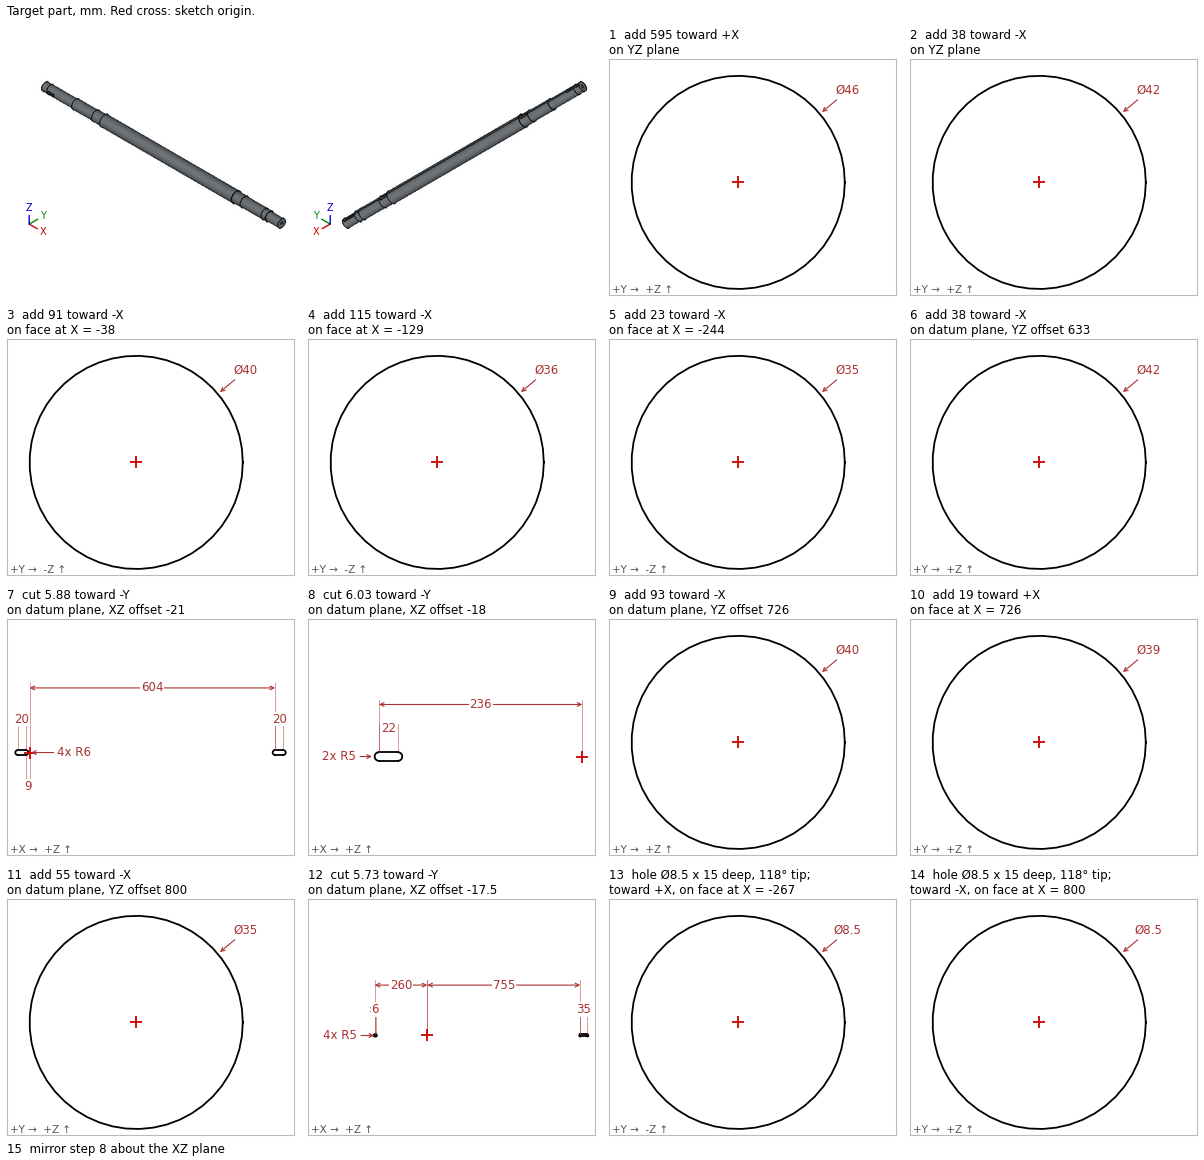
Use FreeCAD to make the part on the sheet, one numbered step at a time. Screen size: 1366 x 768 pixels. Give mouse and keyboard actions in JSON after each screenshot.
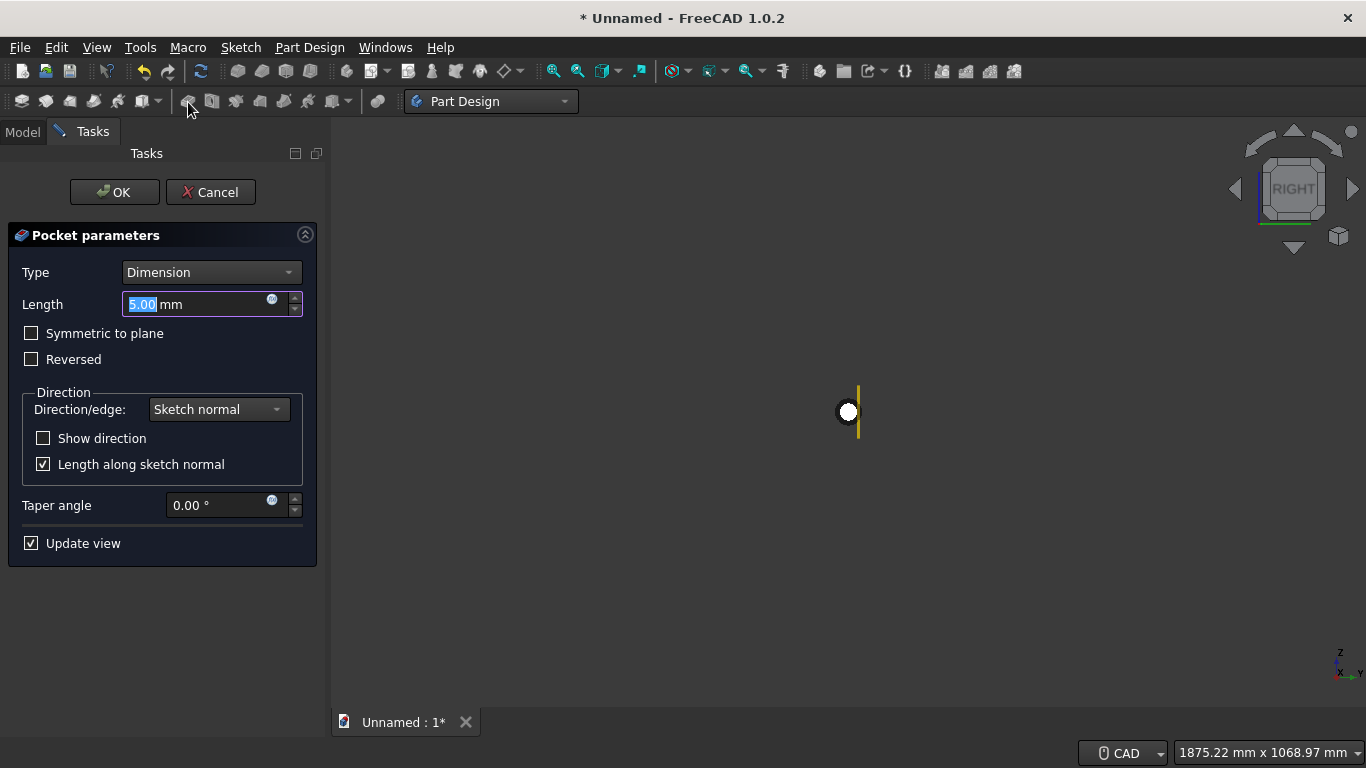
{"action": "type", "text": "5.73"}
{"action": "key", "text": "Tab"}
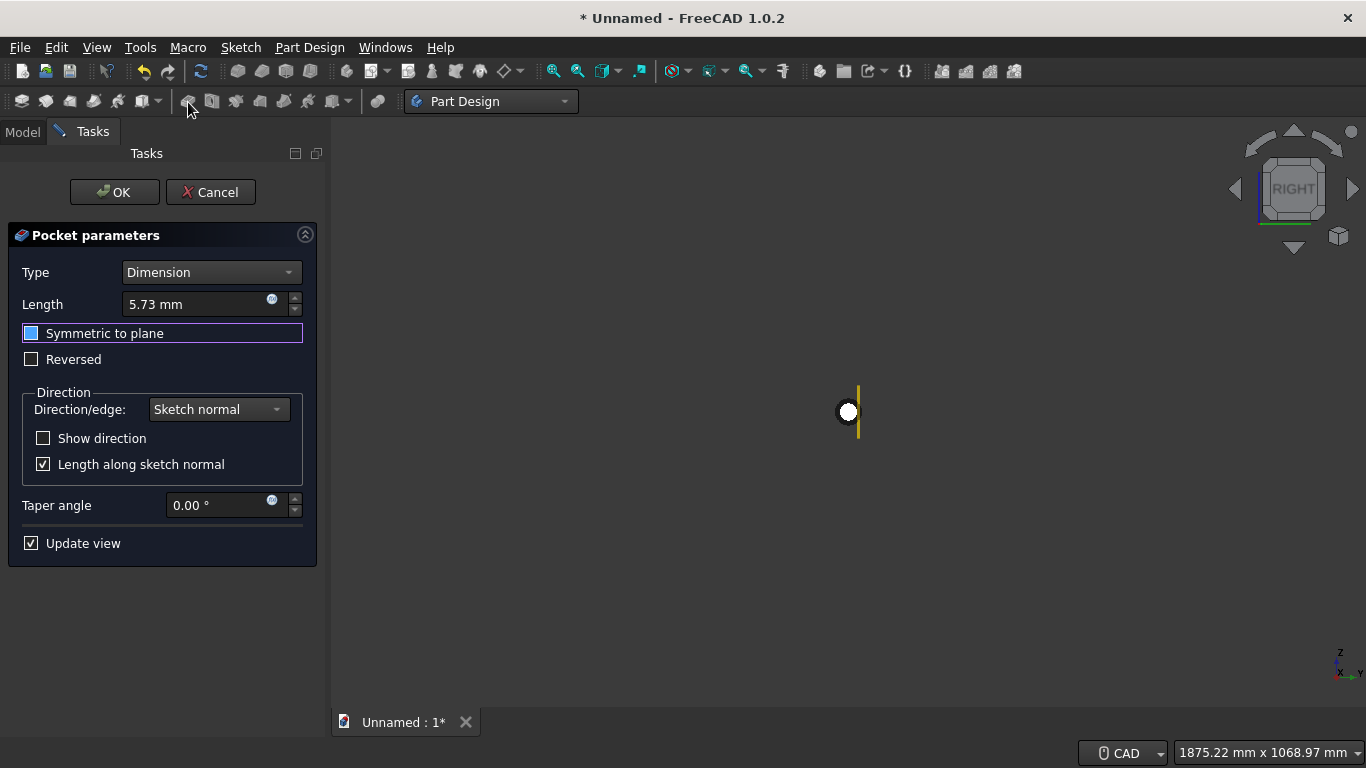
{"action": "left_click", "coordinate": [30, 359]}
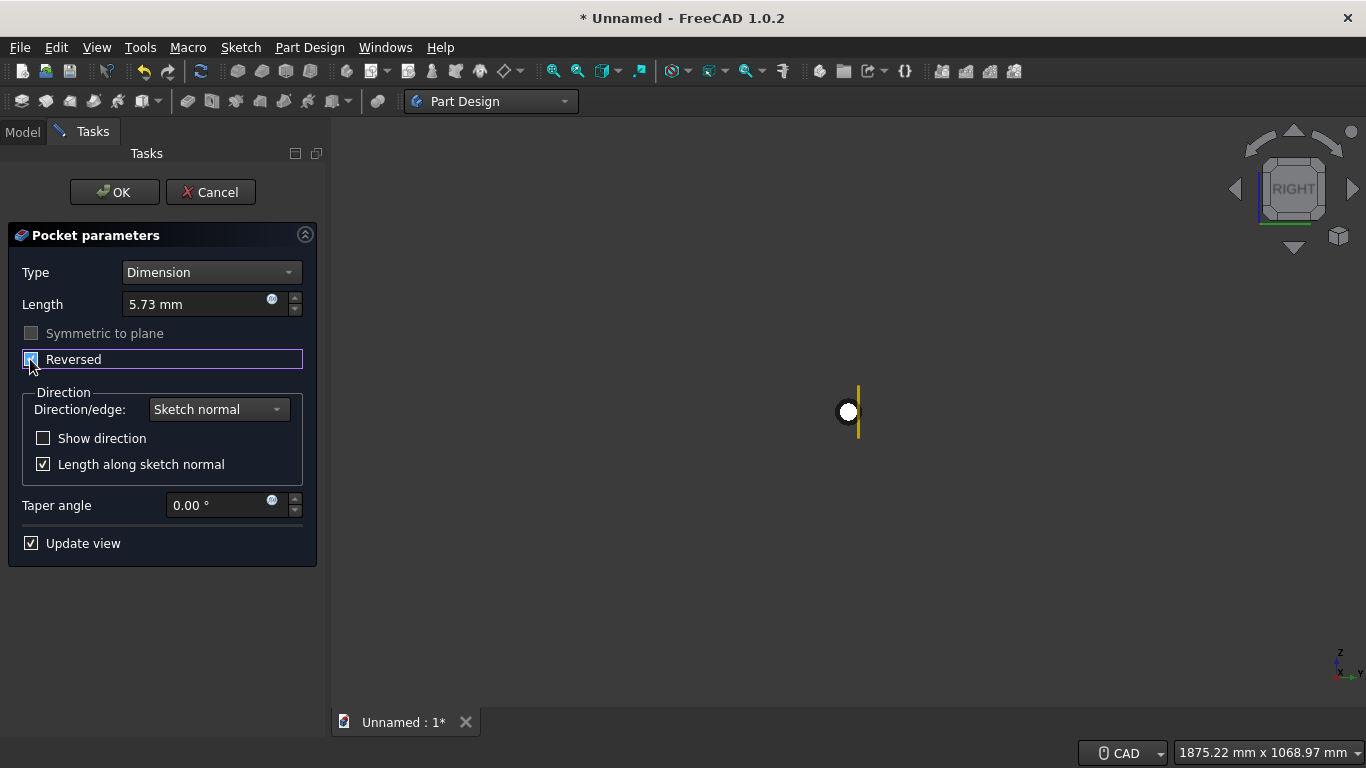
{"action": "left_click", "coordinate": [115, 192]}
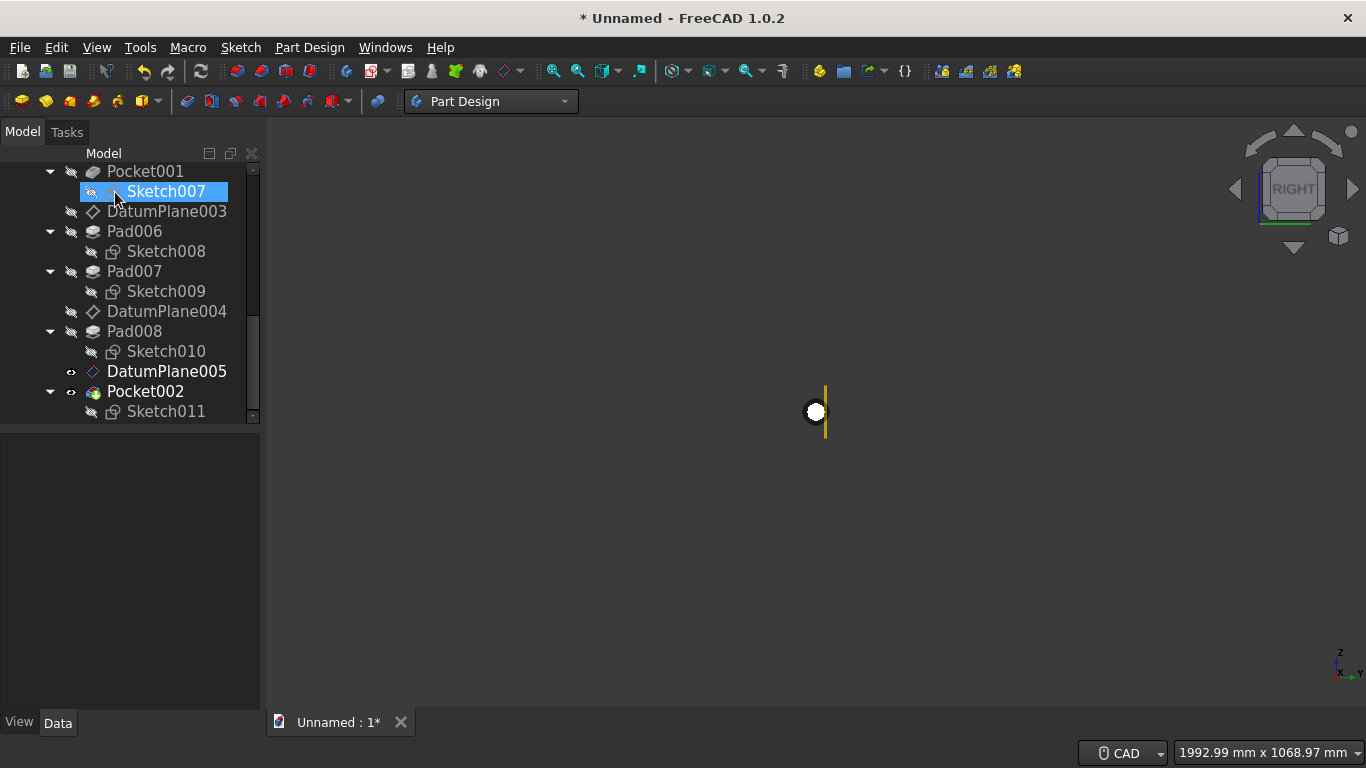
{"action": "left_click", "coordinate": [116, 372]}
{"action": "key", "text": "space"}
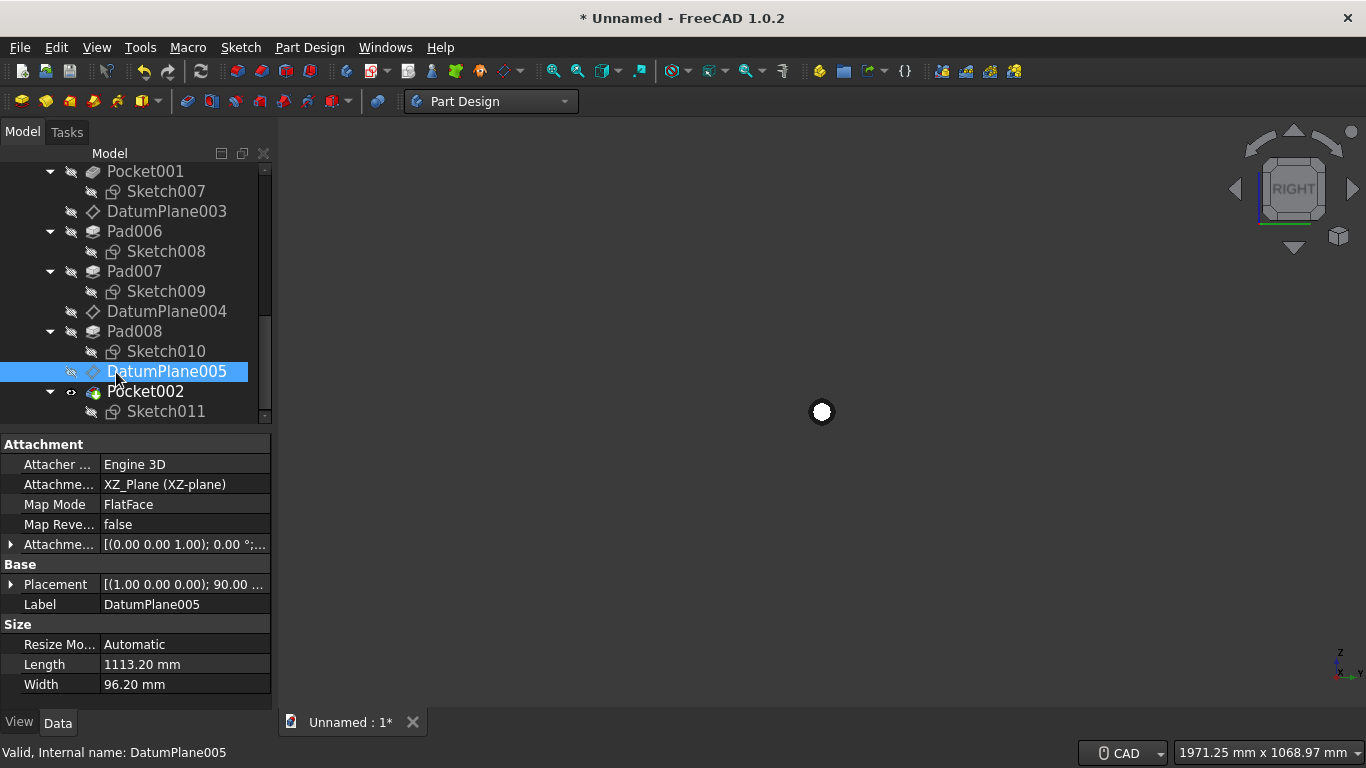
{"action": "key", "text": "v f"}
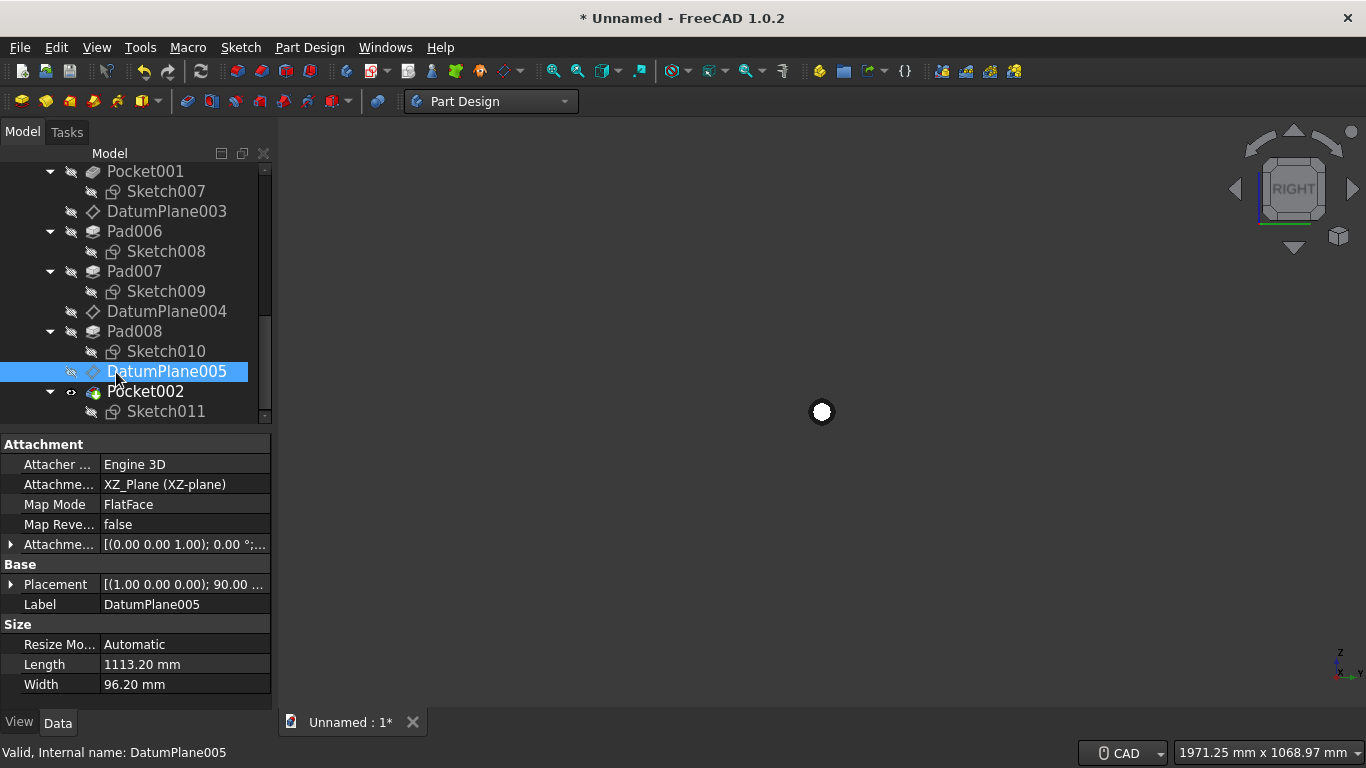
{"action": "key", "text": "6"}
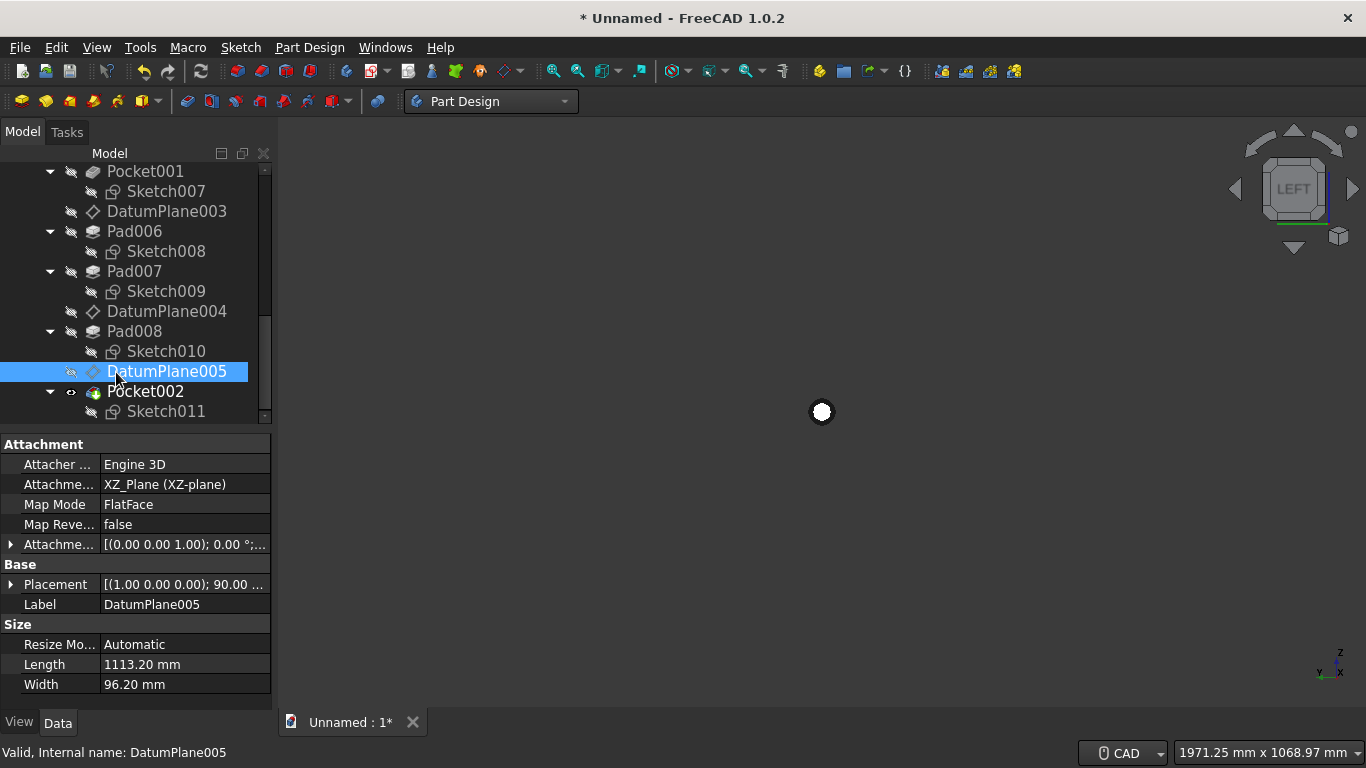
{"action": "key", "text": "v f"}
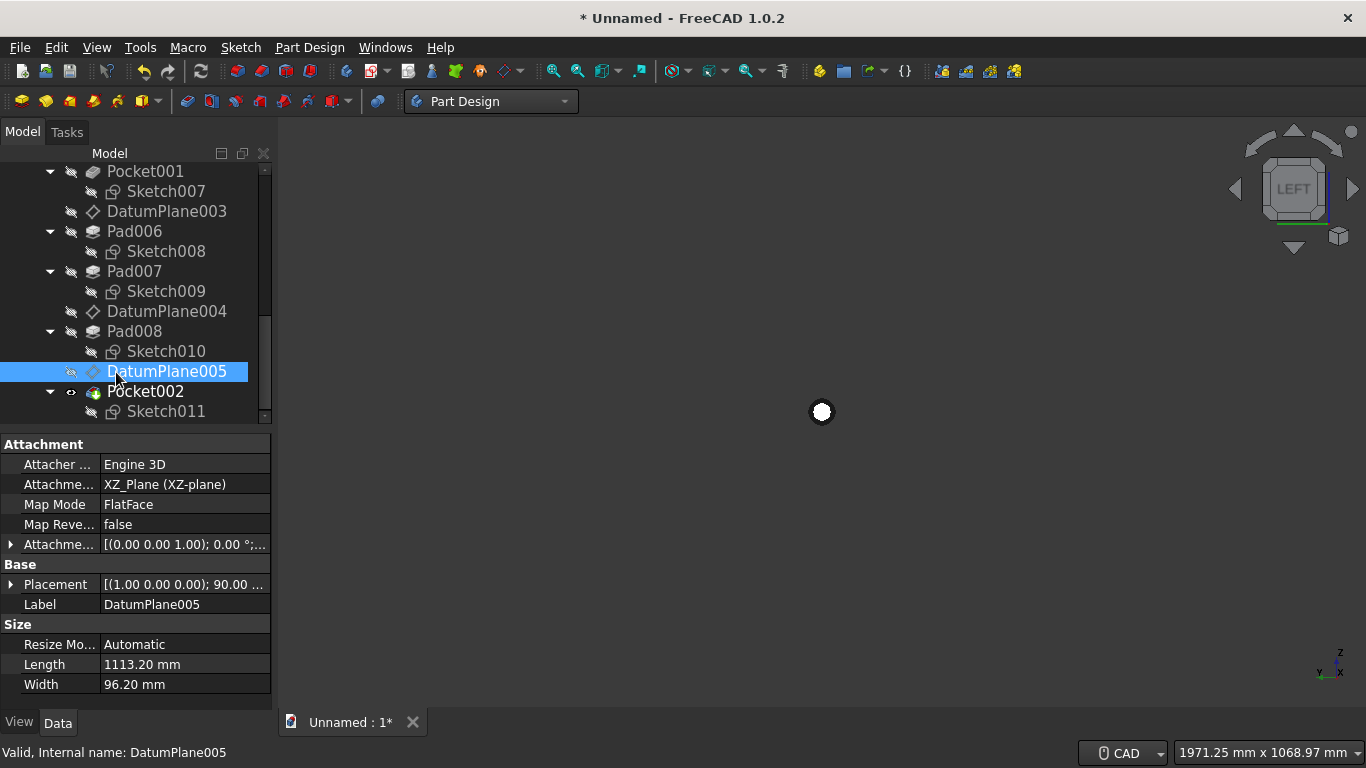
{"action": "left_click", "coordinate": [822, 411]}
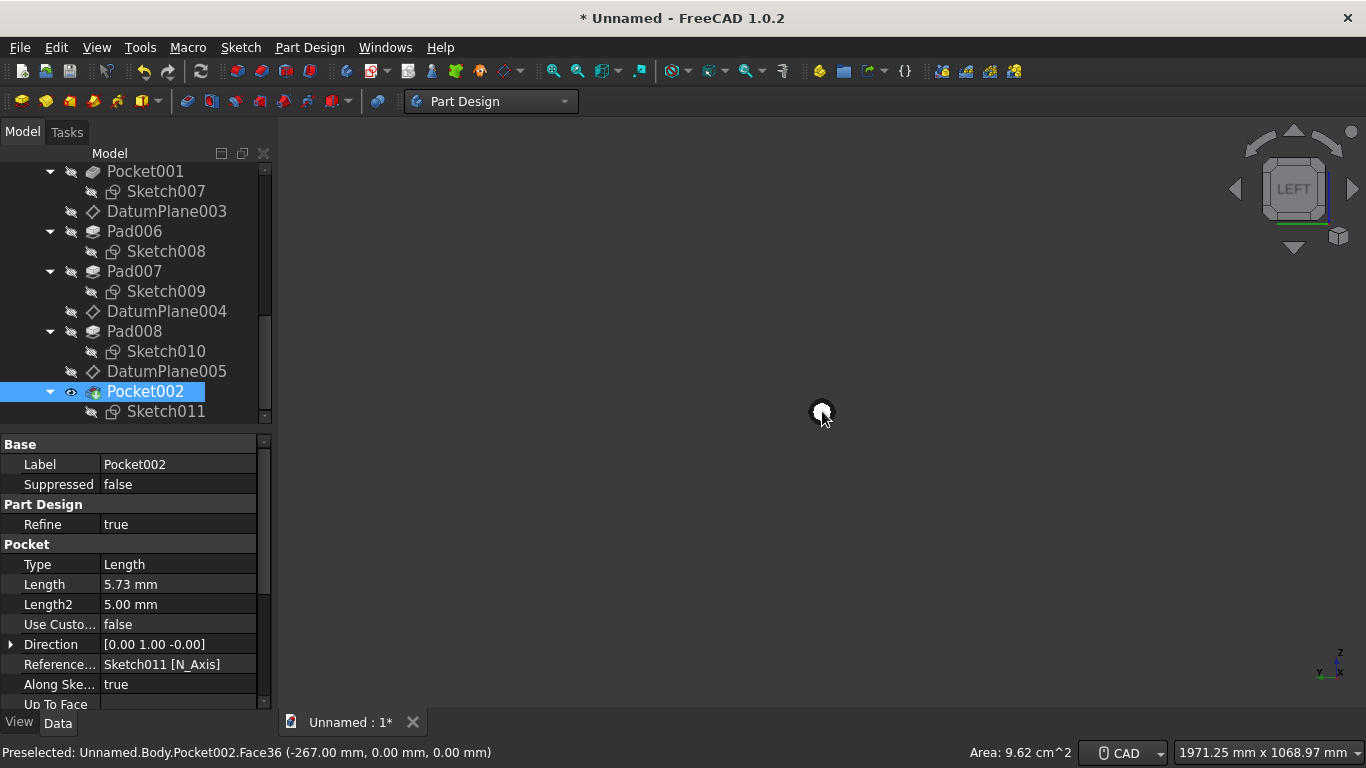
{"action": "left_click", "coordinate": [372, 72]}